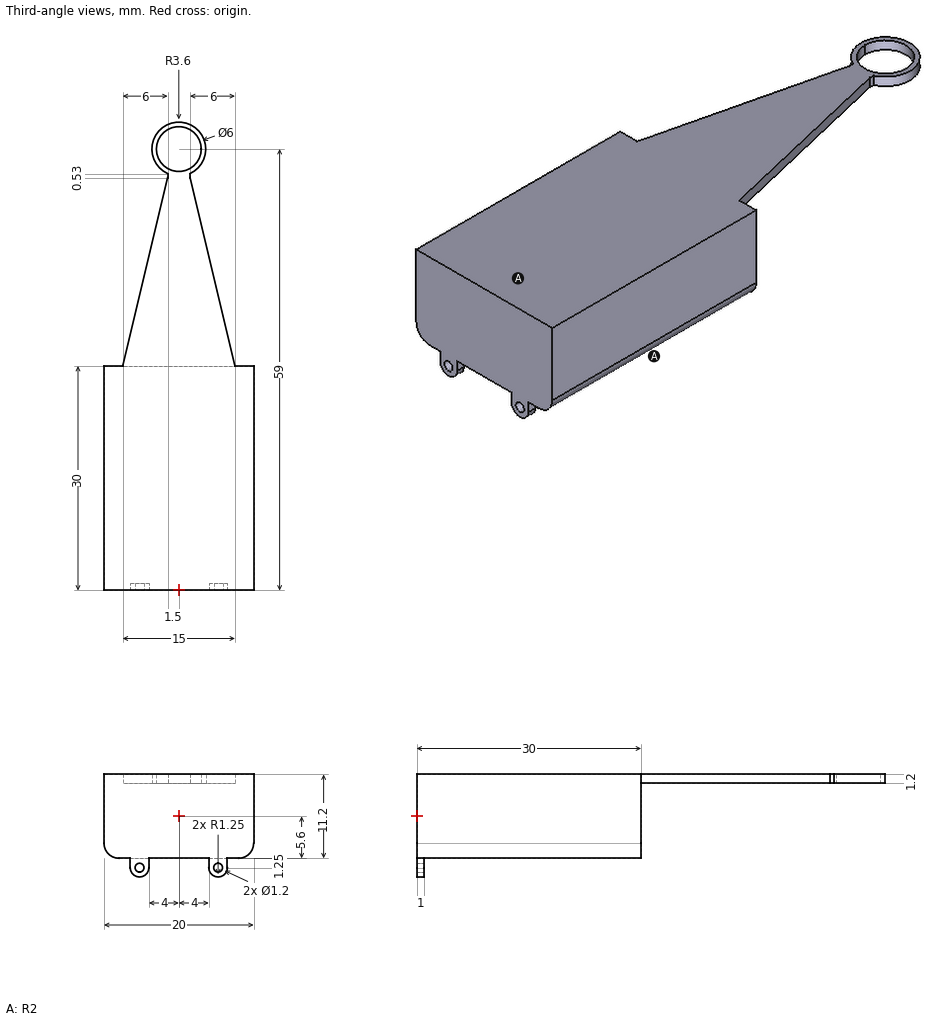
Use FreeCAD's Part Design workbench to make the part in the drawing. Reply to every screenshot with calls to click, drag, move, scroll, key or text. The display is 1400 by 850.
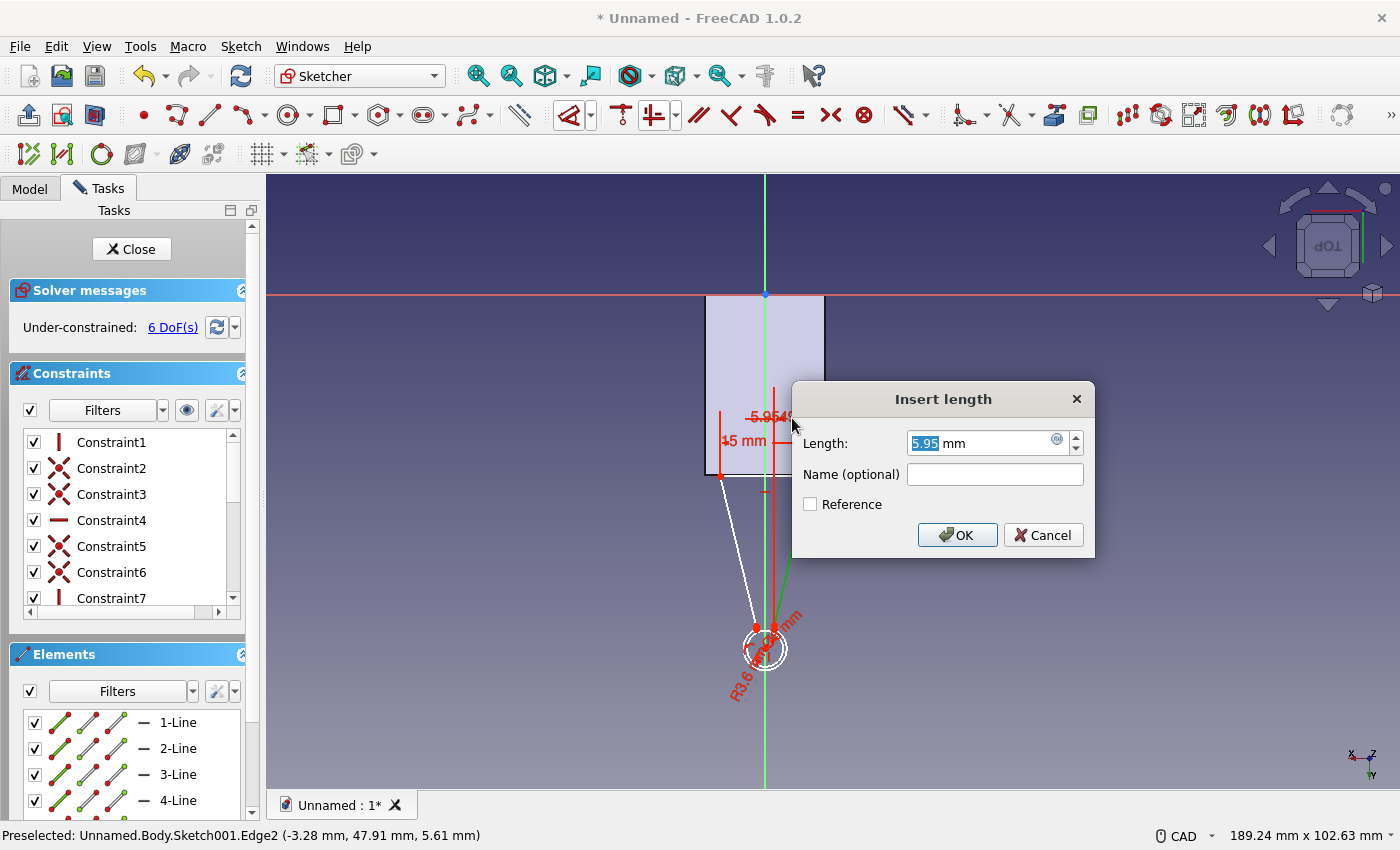
text(6)
key(Return)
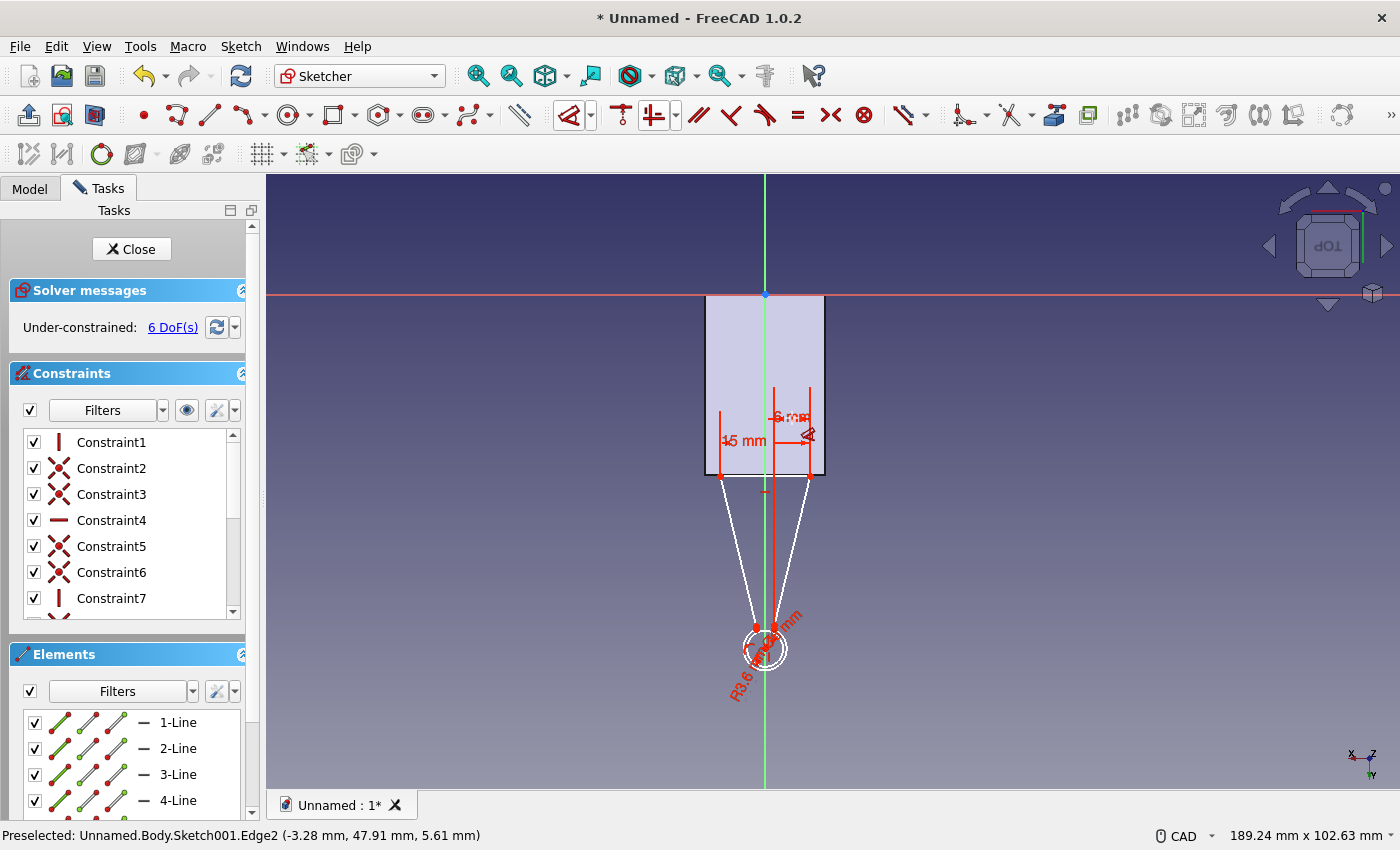
click(731, 521)
click(738, 708)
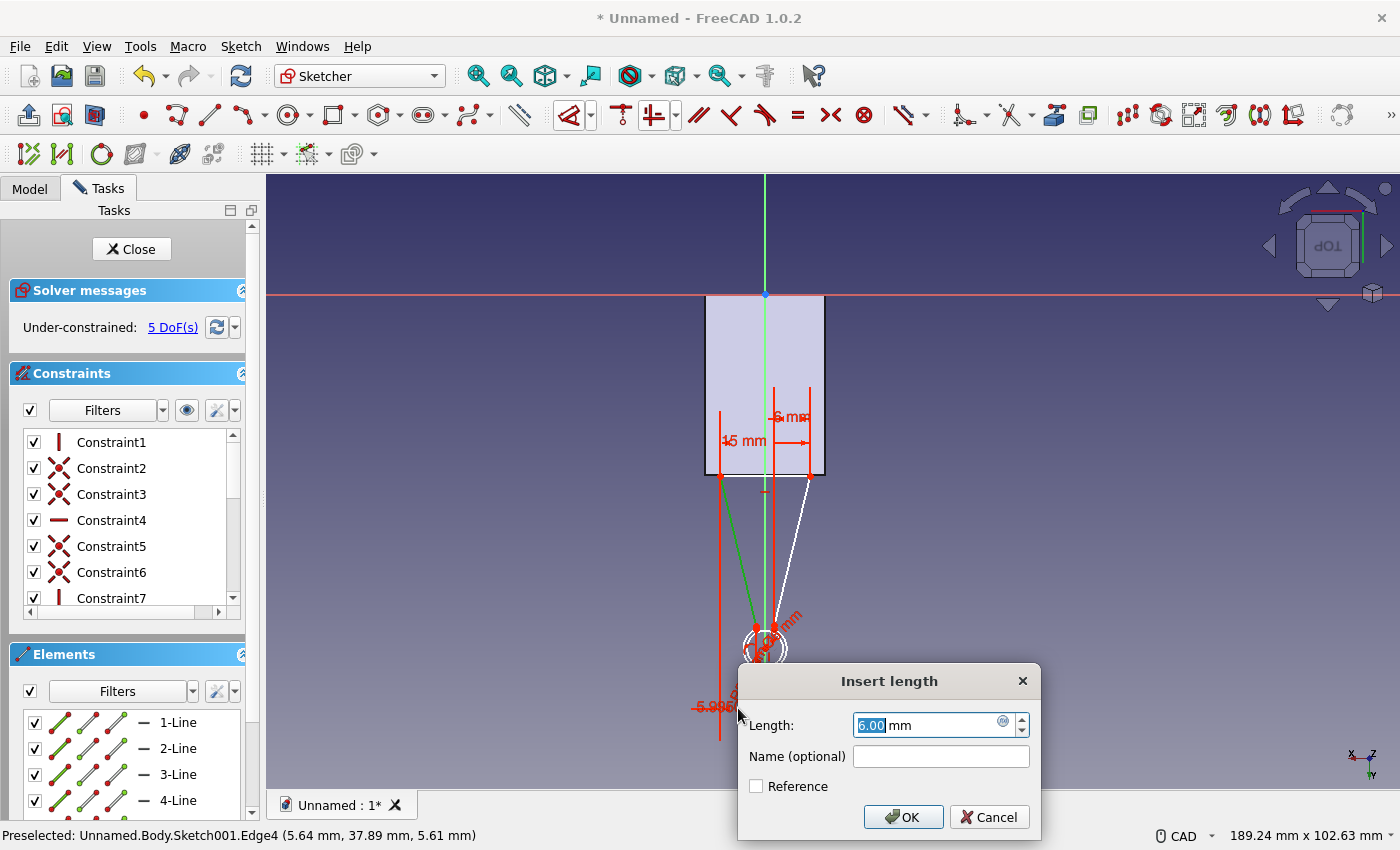
text(6)
key(Return)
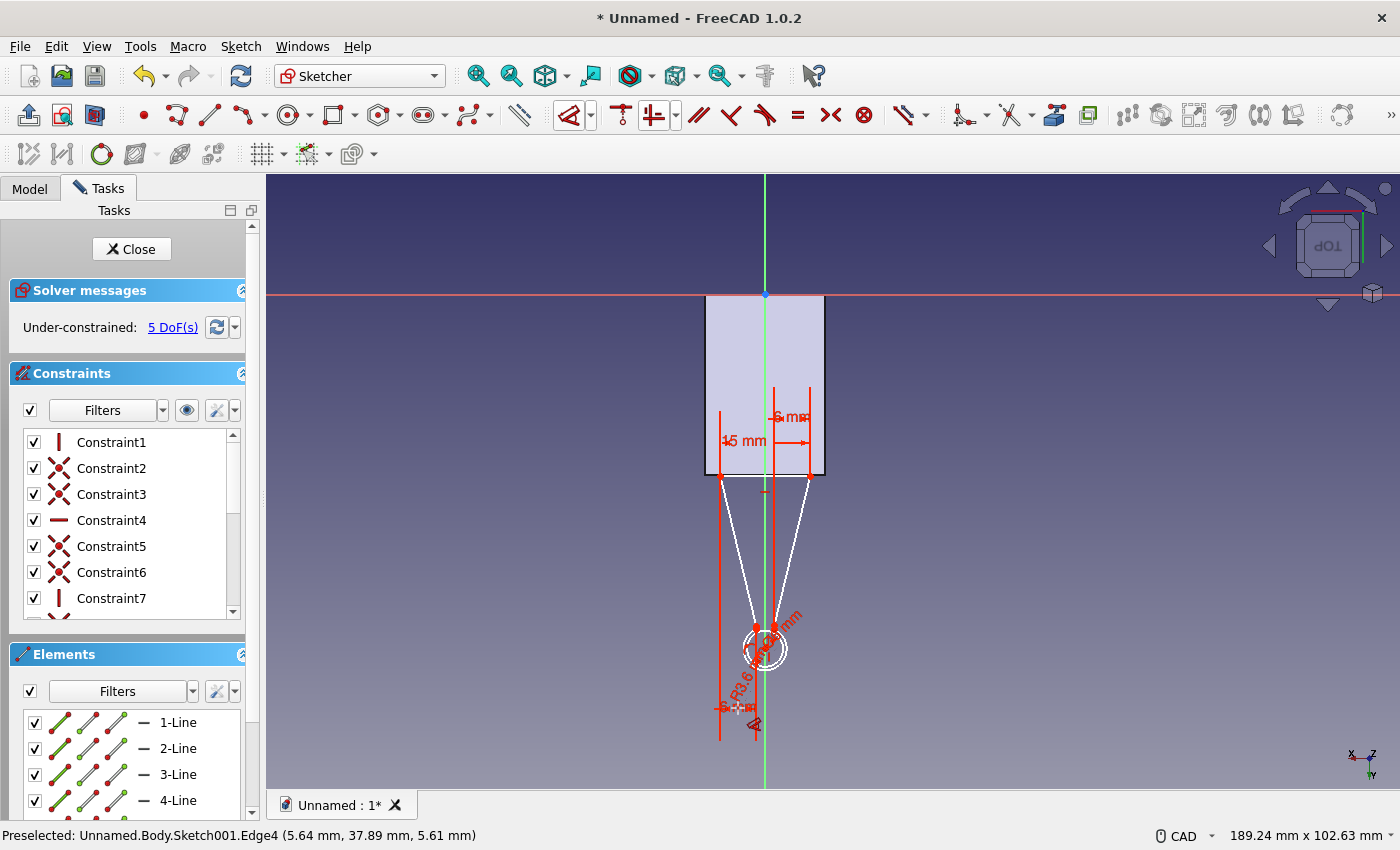
click(765, 649)
click(799, 390)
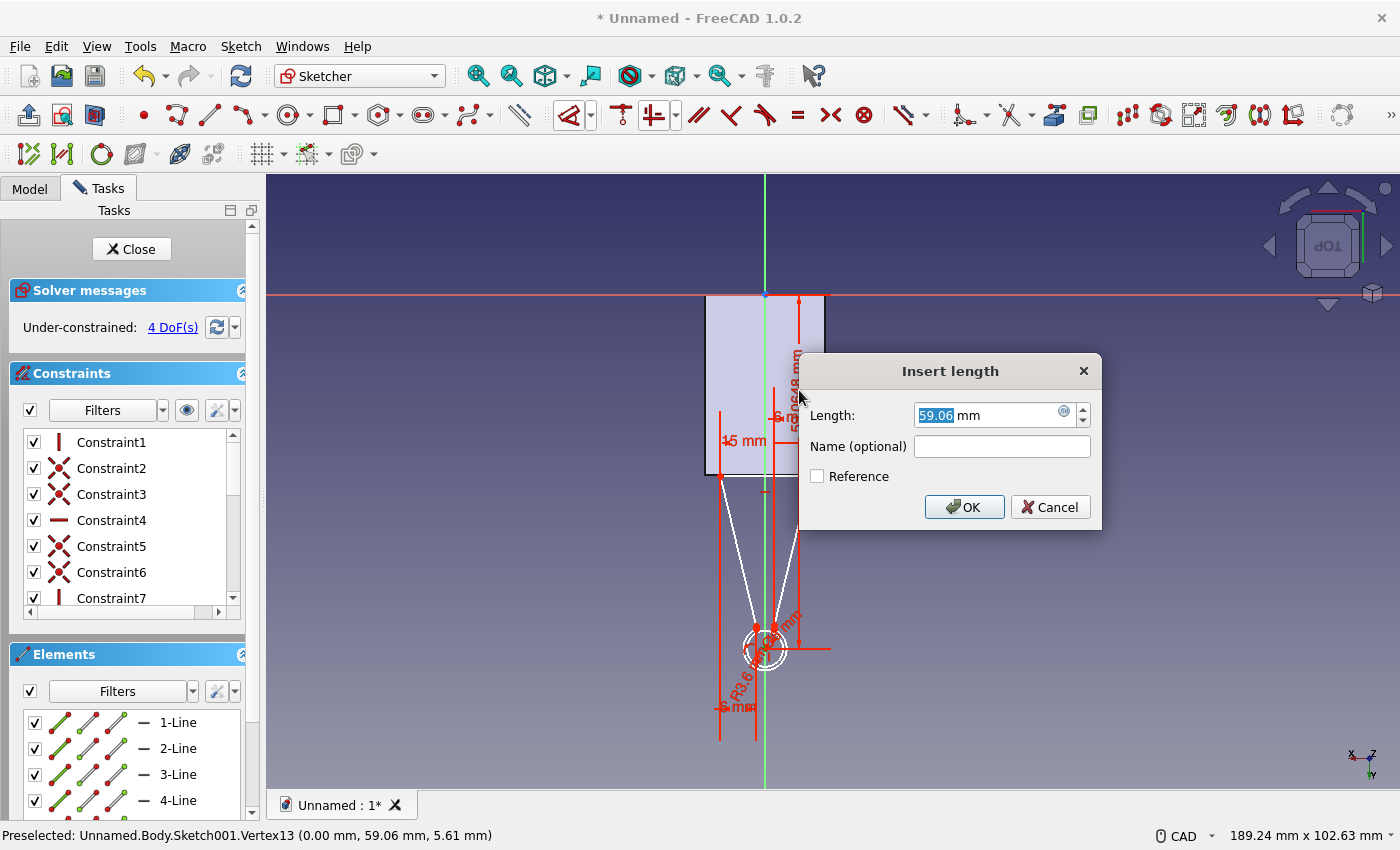
text(59)
key(Return)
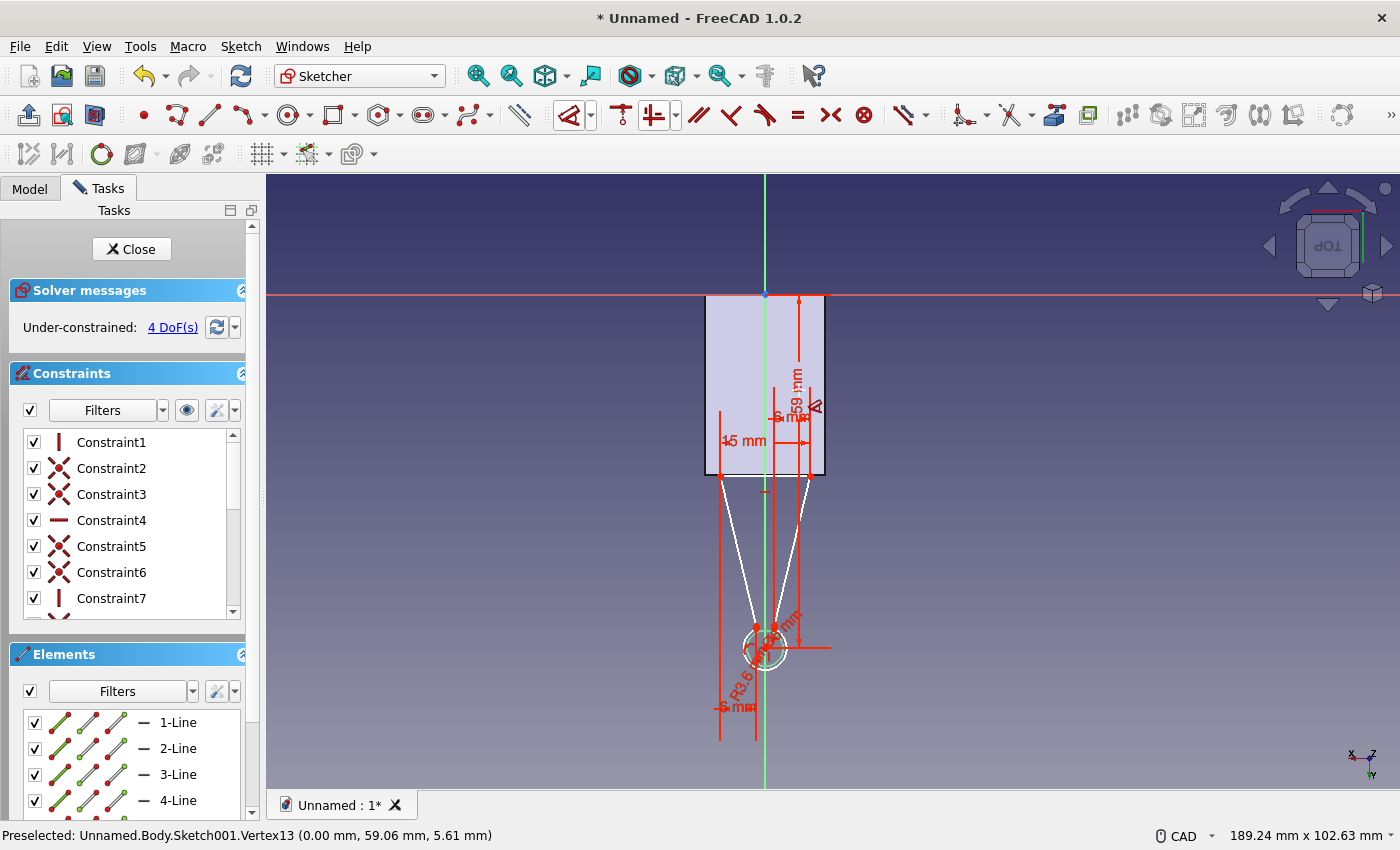
click(810, 476)
click(844, 344)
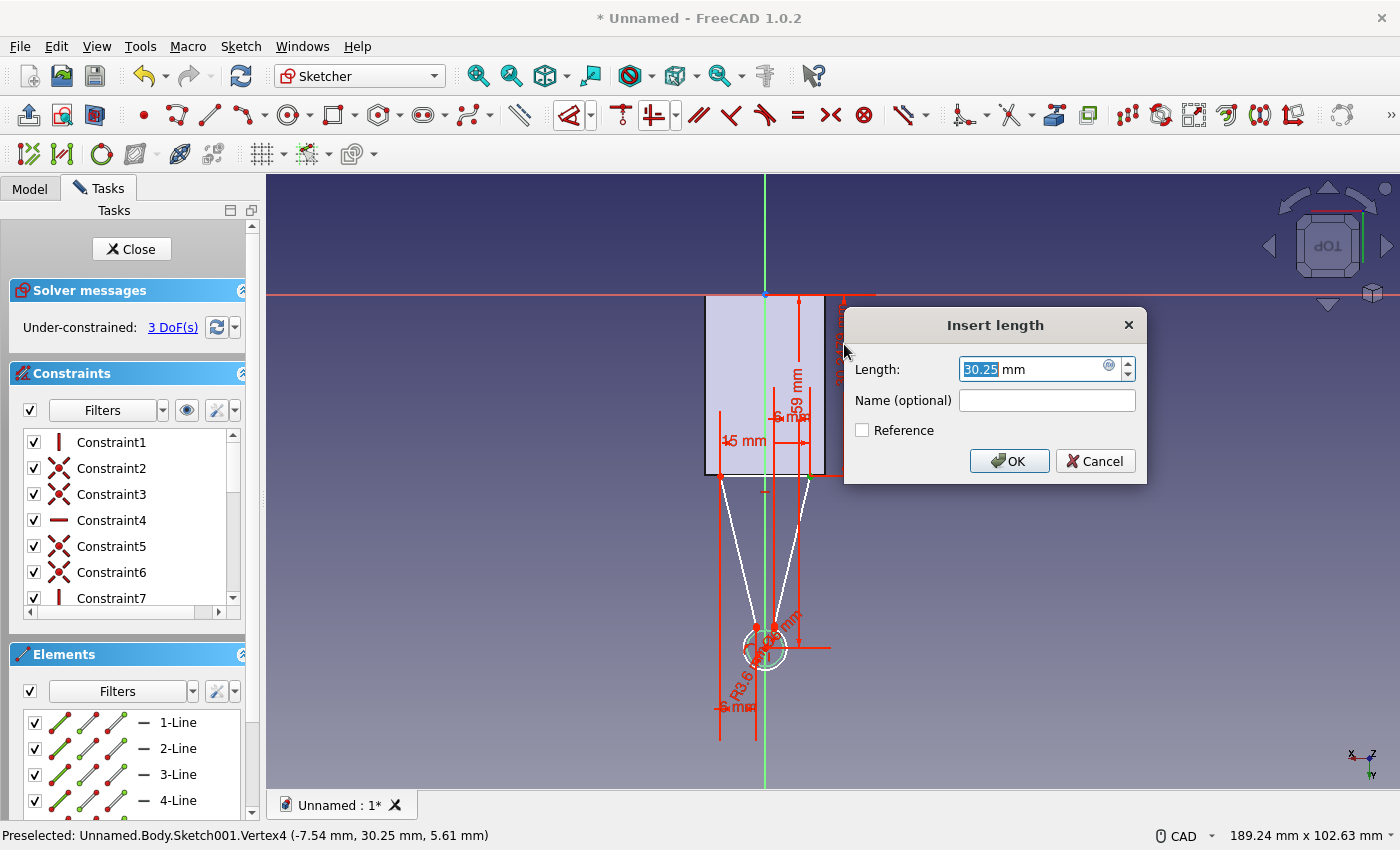
text(30)
key(Return)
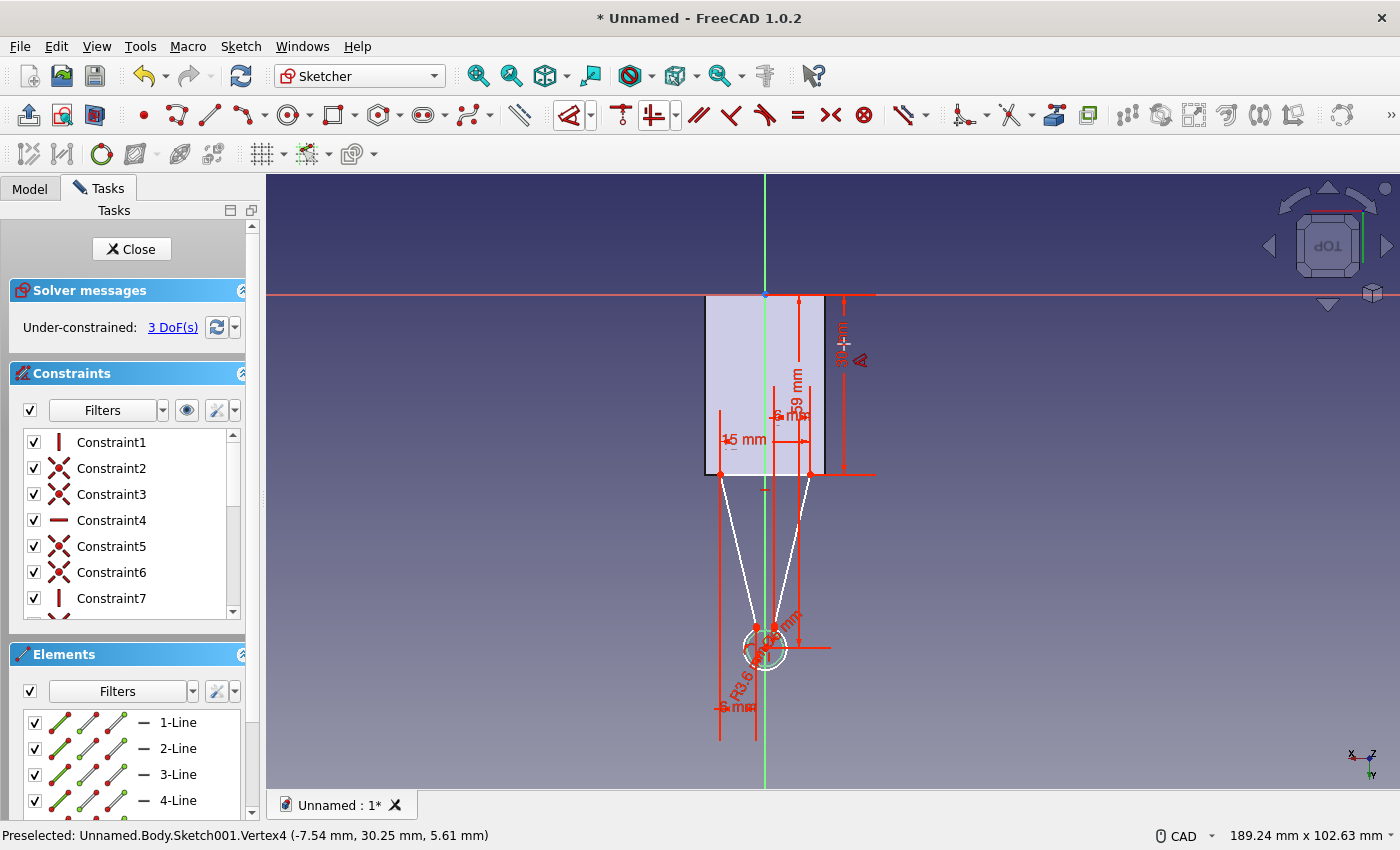
scroll(774, 627, up, 13)